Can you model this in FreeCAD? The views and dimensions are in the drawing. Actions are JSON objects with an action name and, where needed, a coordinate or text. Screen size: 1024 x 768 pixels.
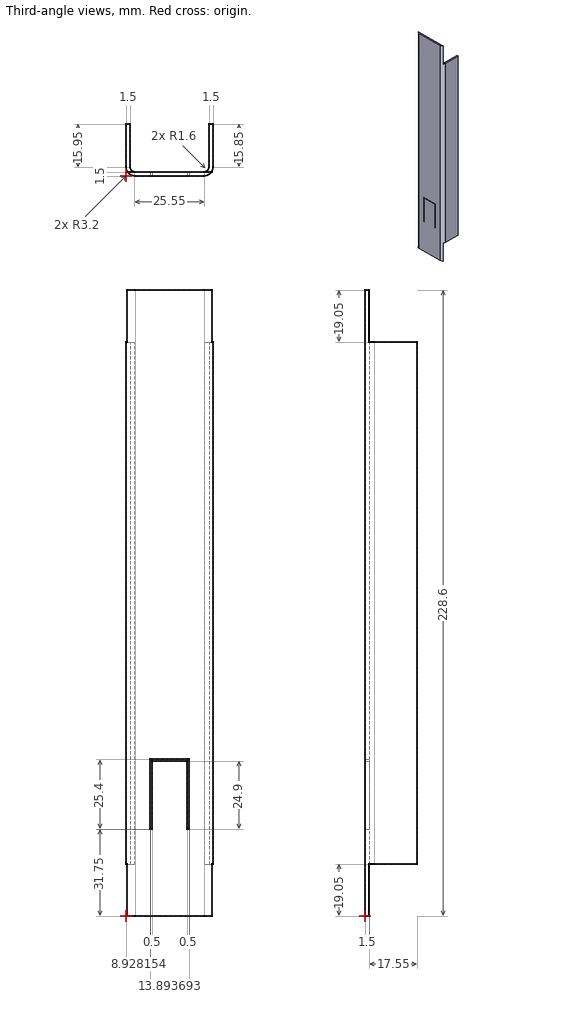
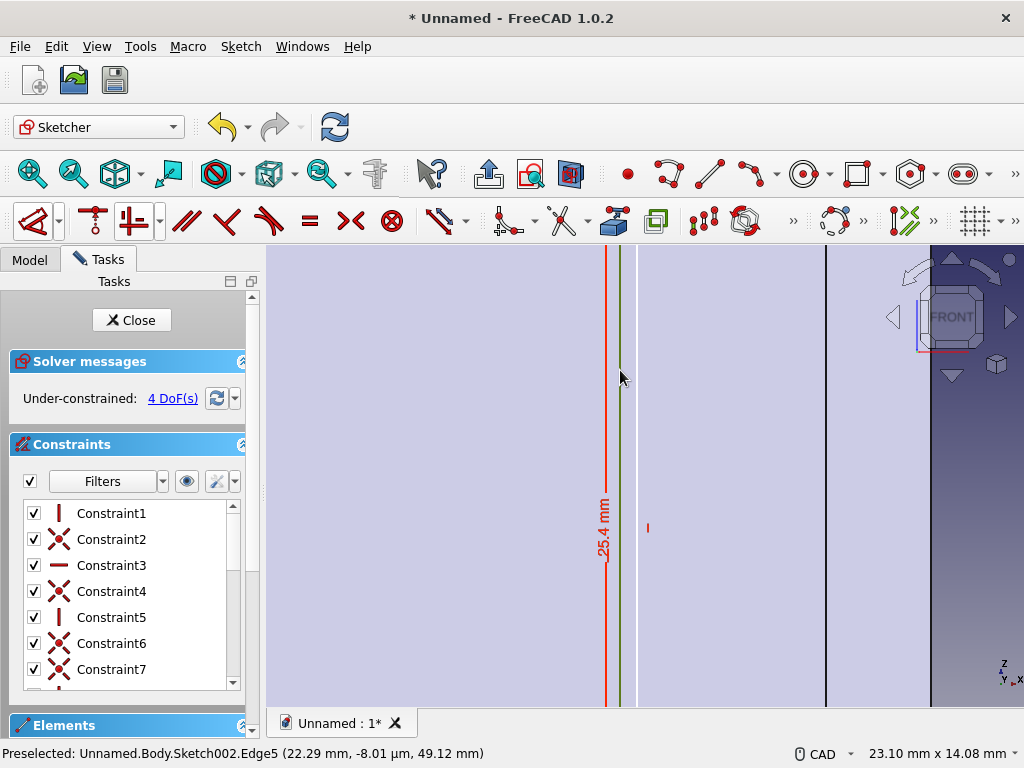
{"action": "left_click", "coordinate": [58, 222]}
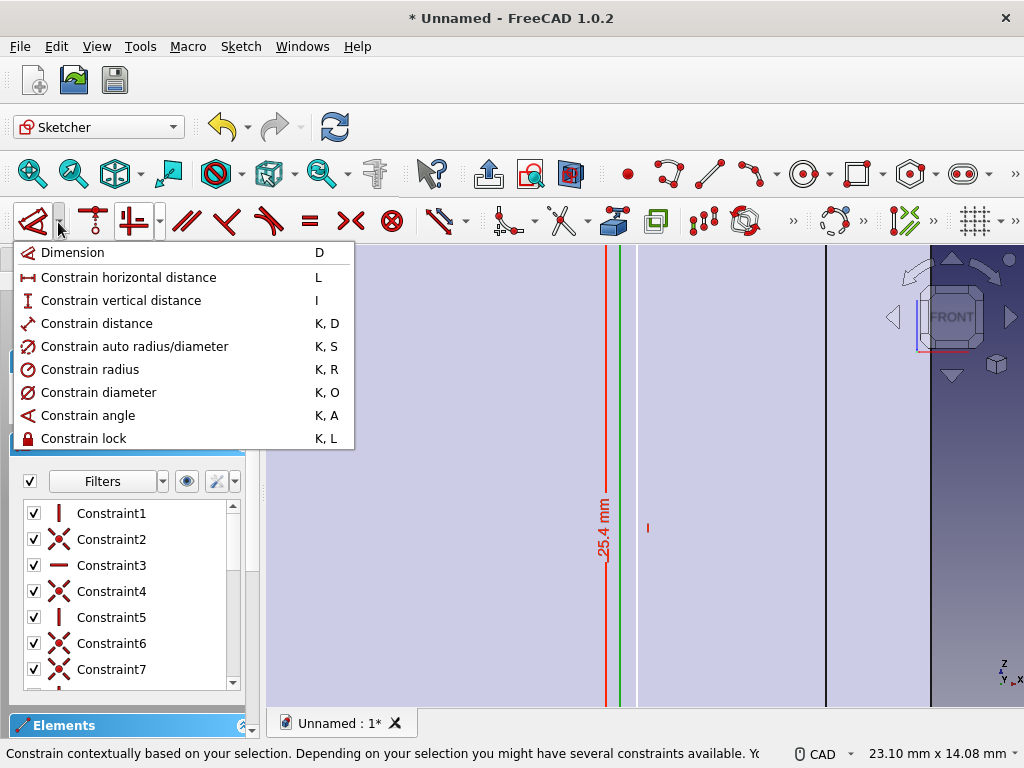
{"action": "left_click", "coordinate": [184, 300]}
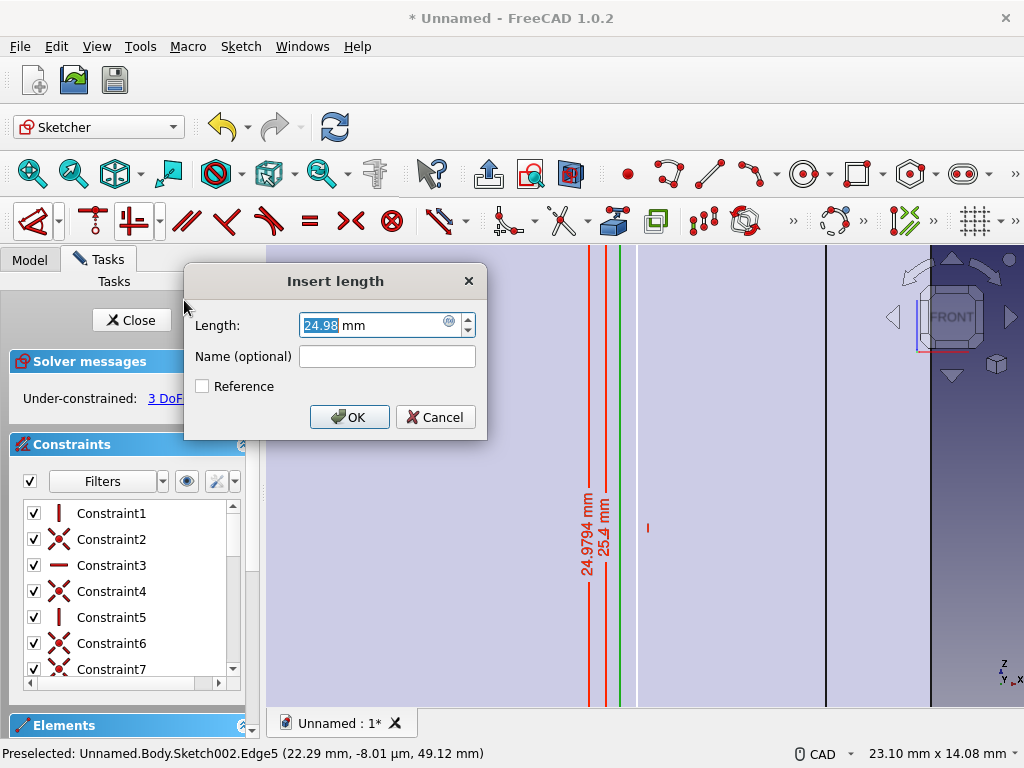
{"action": "type", "text": "24.9"}
{"action": "key", "text": "Return"}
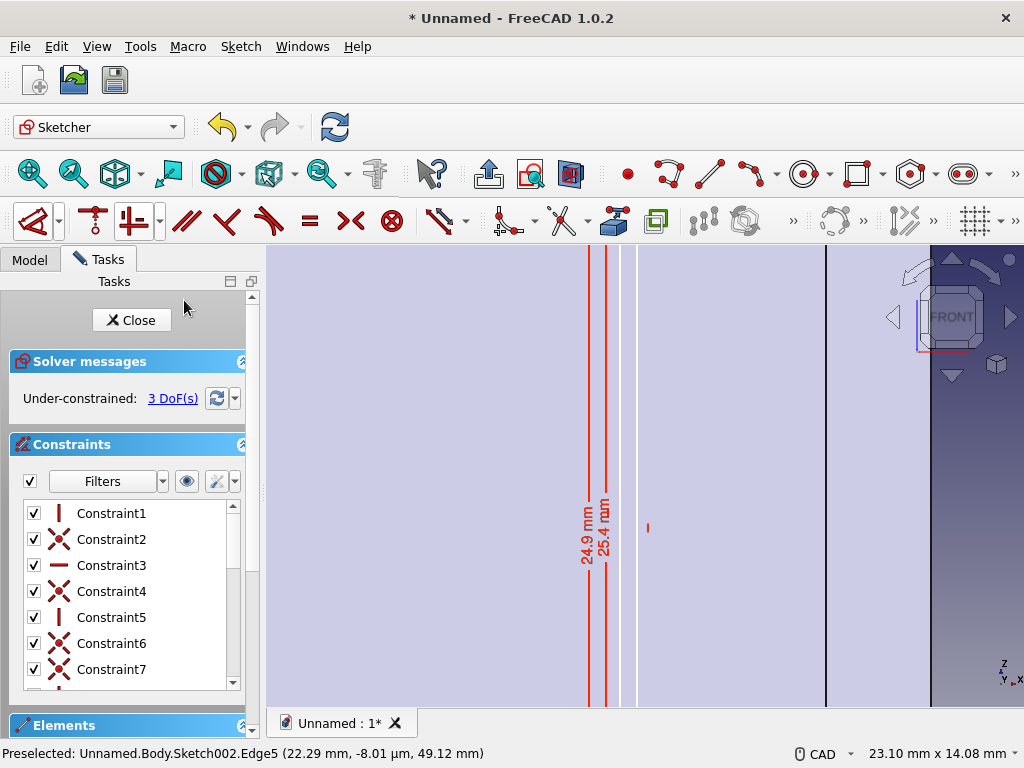
{"action": "scroll", "coordinate": [638, 363], "scroll_direction": "down", "scroll_amount": 9}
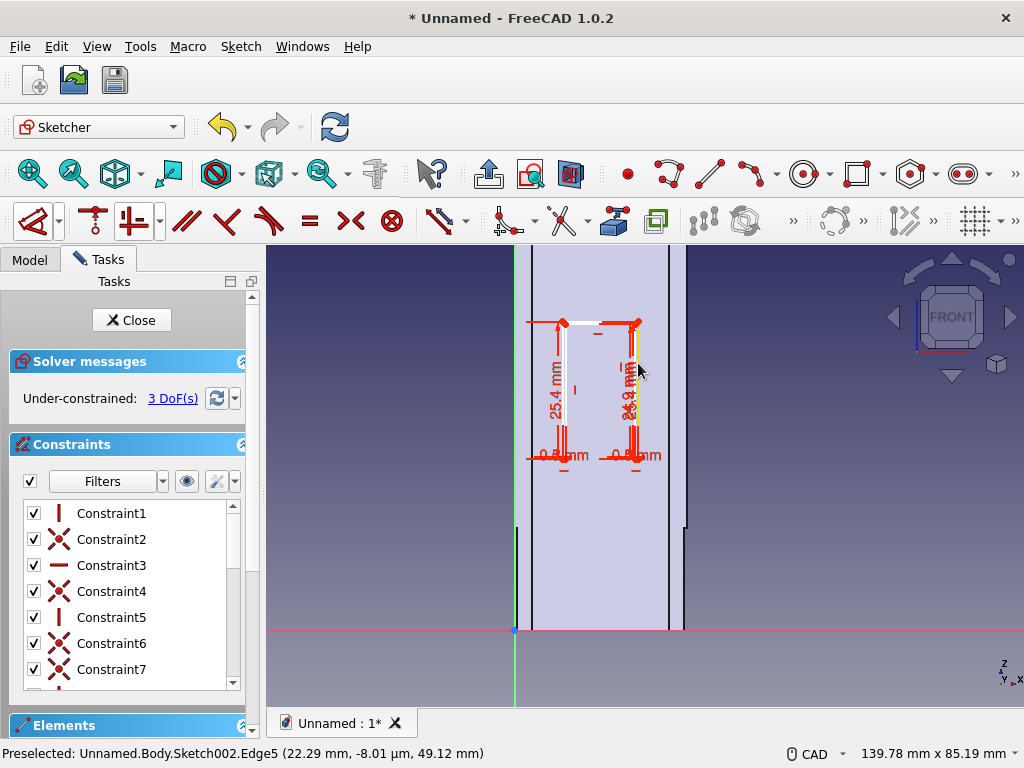
{"action": "scroll", "coordinate": [563, 459], "scroll_direction": "up", "scroll_amount": 8}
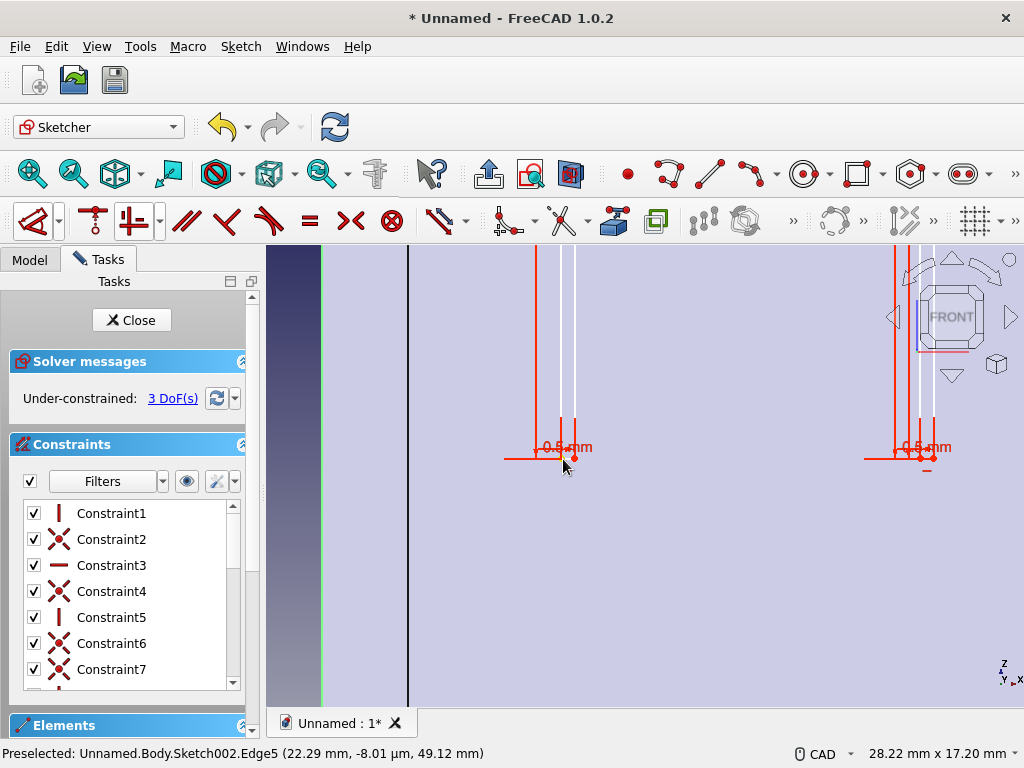
{"action": "left_click", "coordinate": [561, 459]}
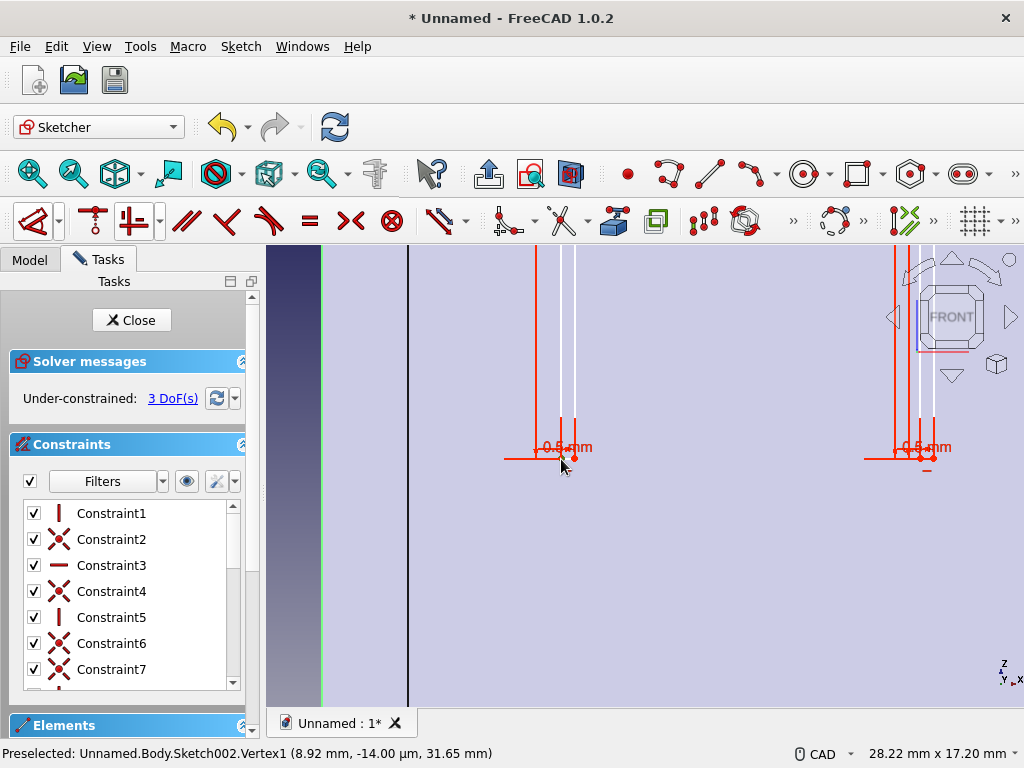
{"action": "key", "text": "i"}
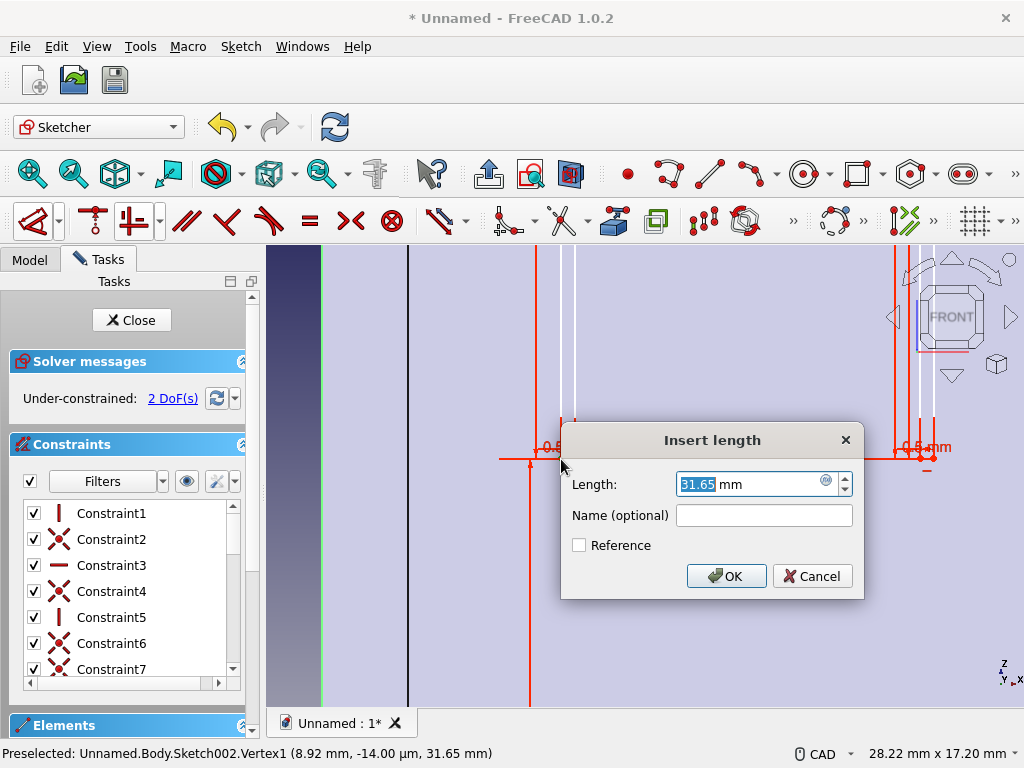
{"action": "type", "text": "31.75"}
{"action": "key", "text": "Return"}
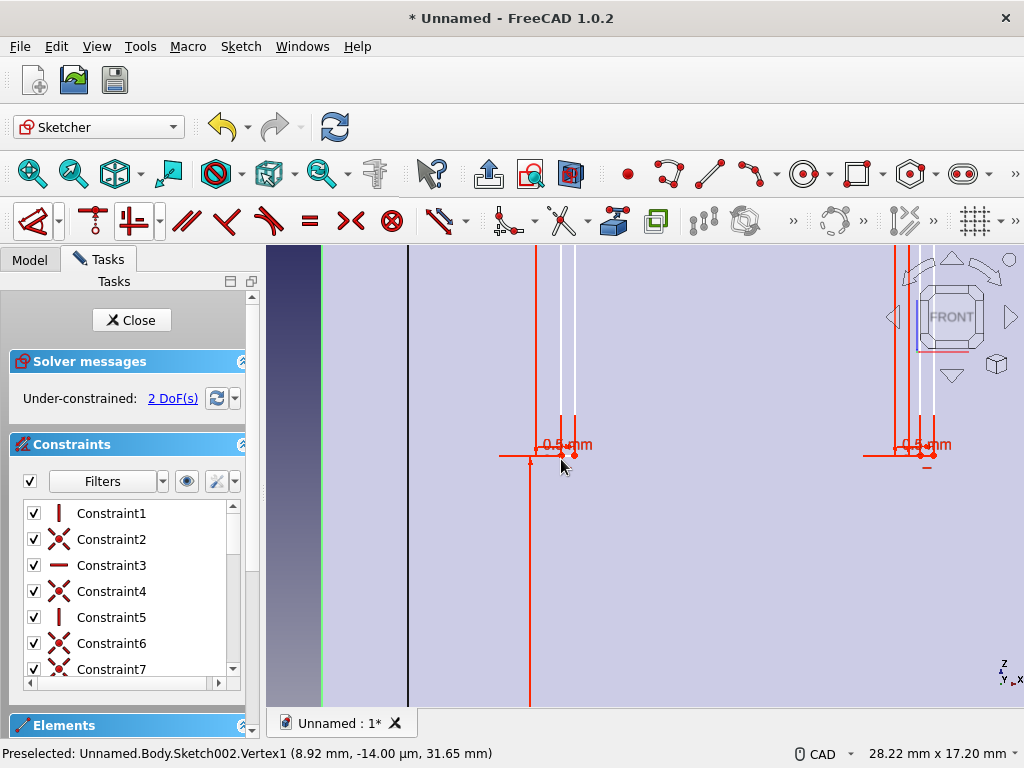
{"action": "scroll", "coordinate": [563, 460], "scroll_direction": "down", "scroll_amount": 8}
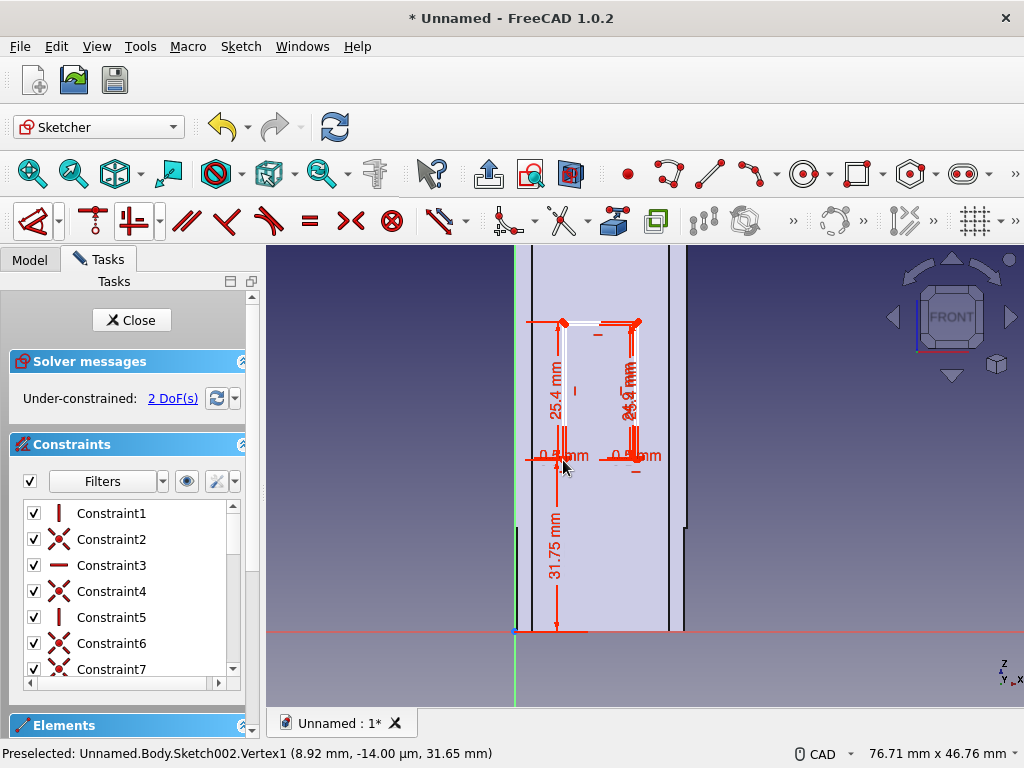
{"action": "scroll", "coordinate": [586, 322], "scroll_direction": "up", "scroll_amount": 9}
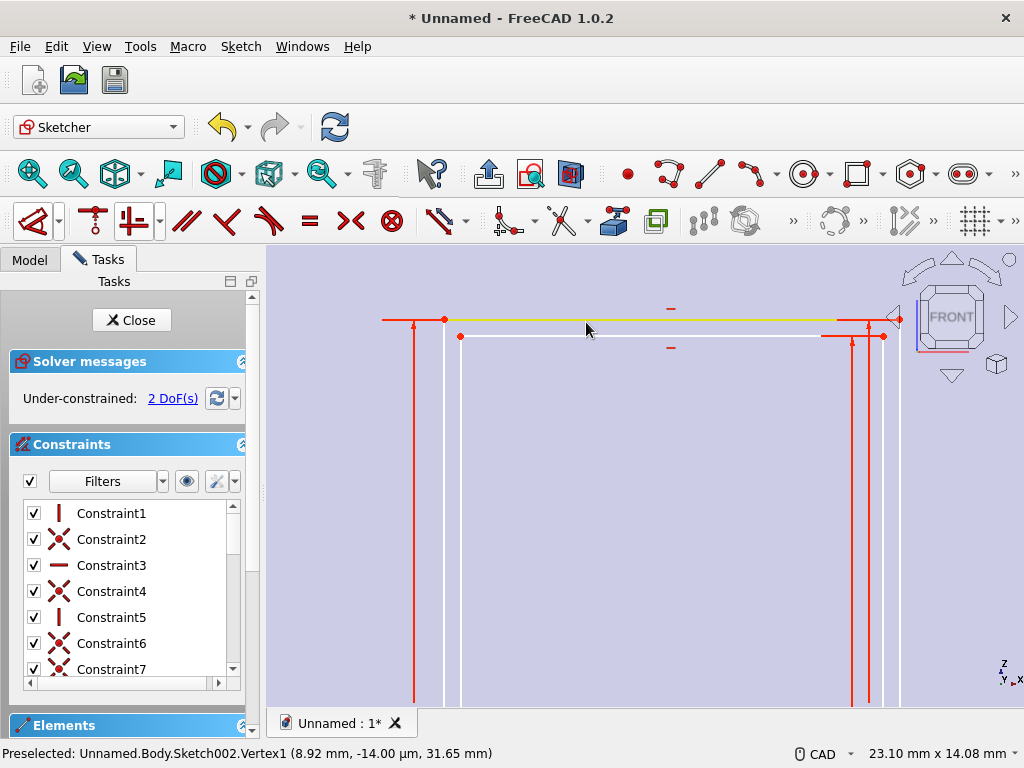
{"action": "left_click", "coordinate": [581, 320]}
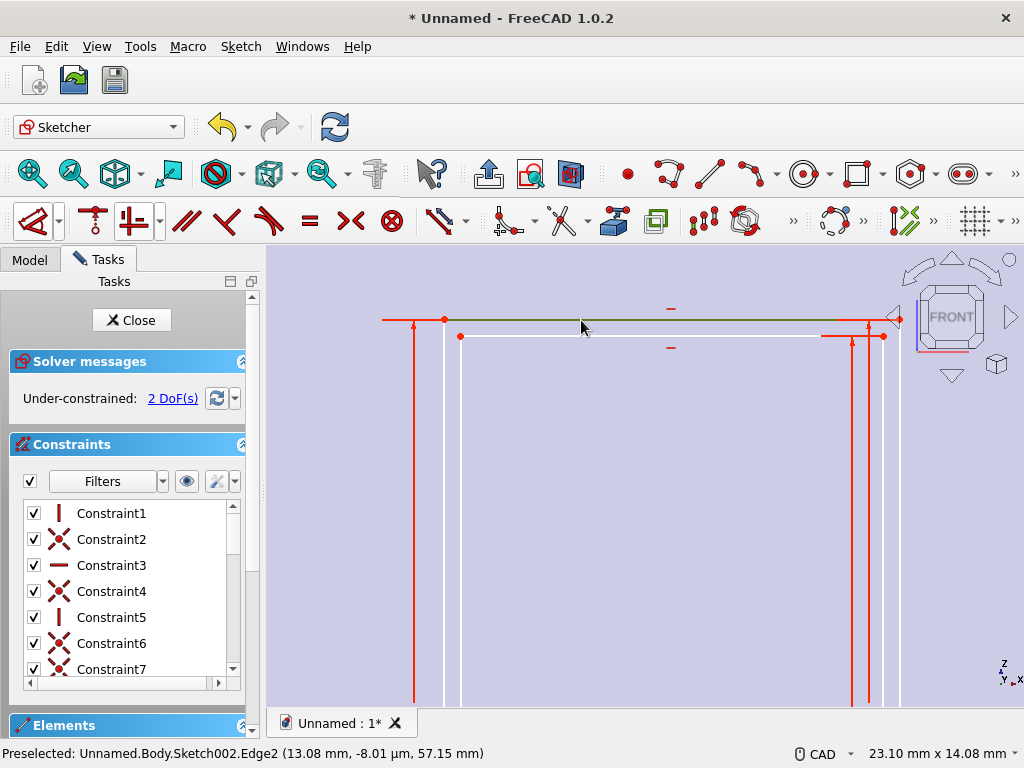
{"action": "left_click", "coordinate": [58, 222]}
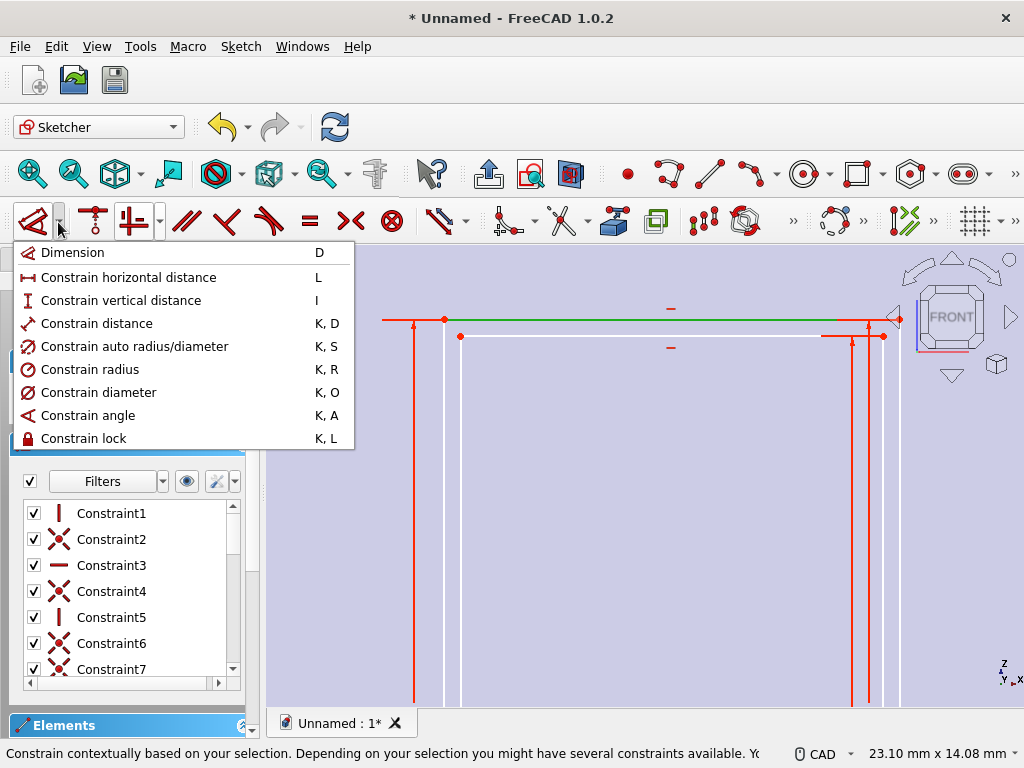
{"action": "left_click", "coordinate": [184, 278]}